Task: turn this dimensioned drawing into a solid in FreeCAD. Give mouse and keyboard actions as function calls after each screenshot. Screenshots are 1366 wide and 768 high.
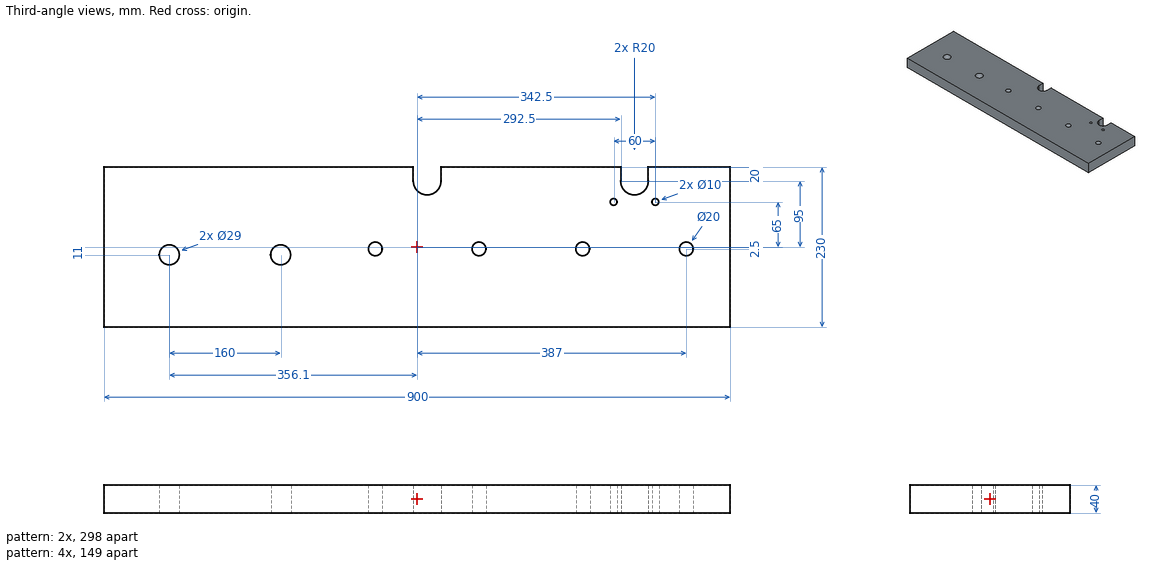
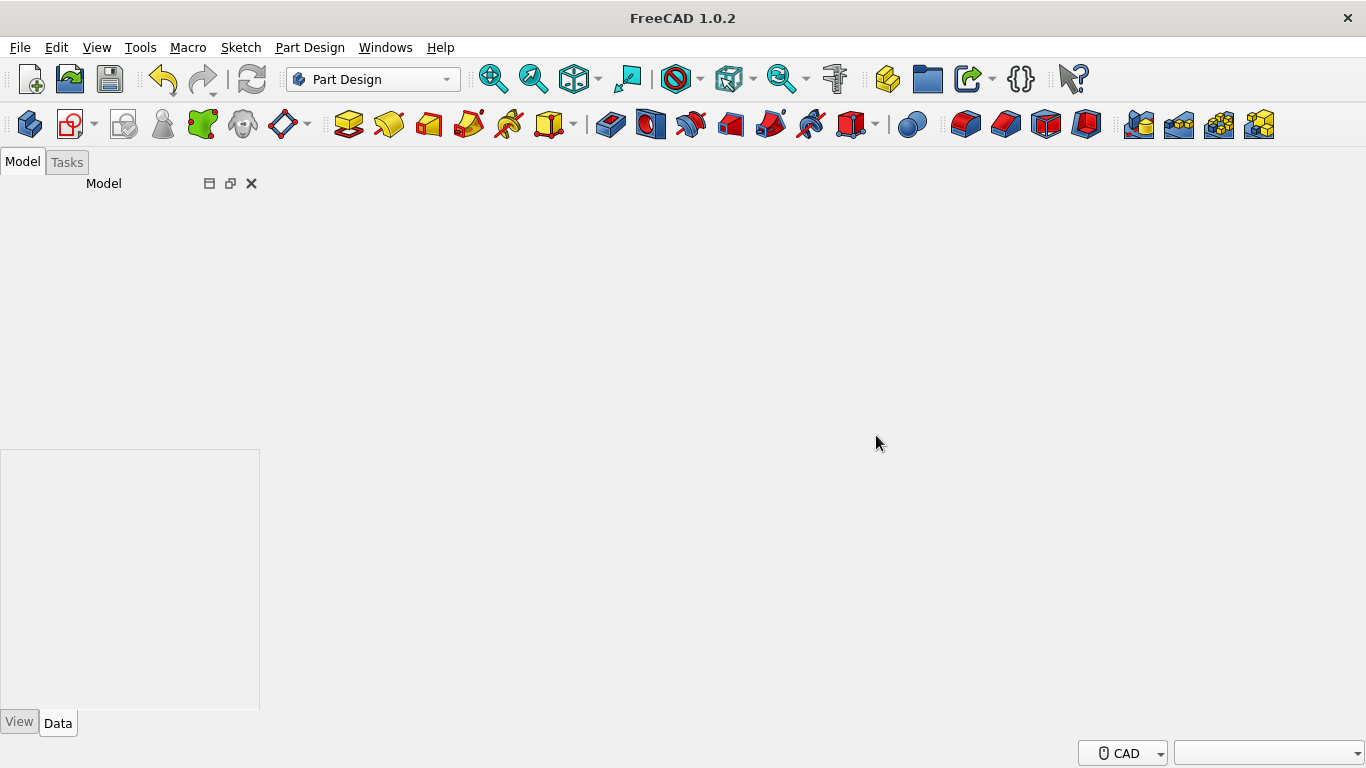
click(30, 80)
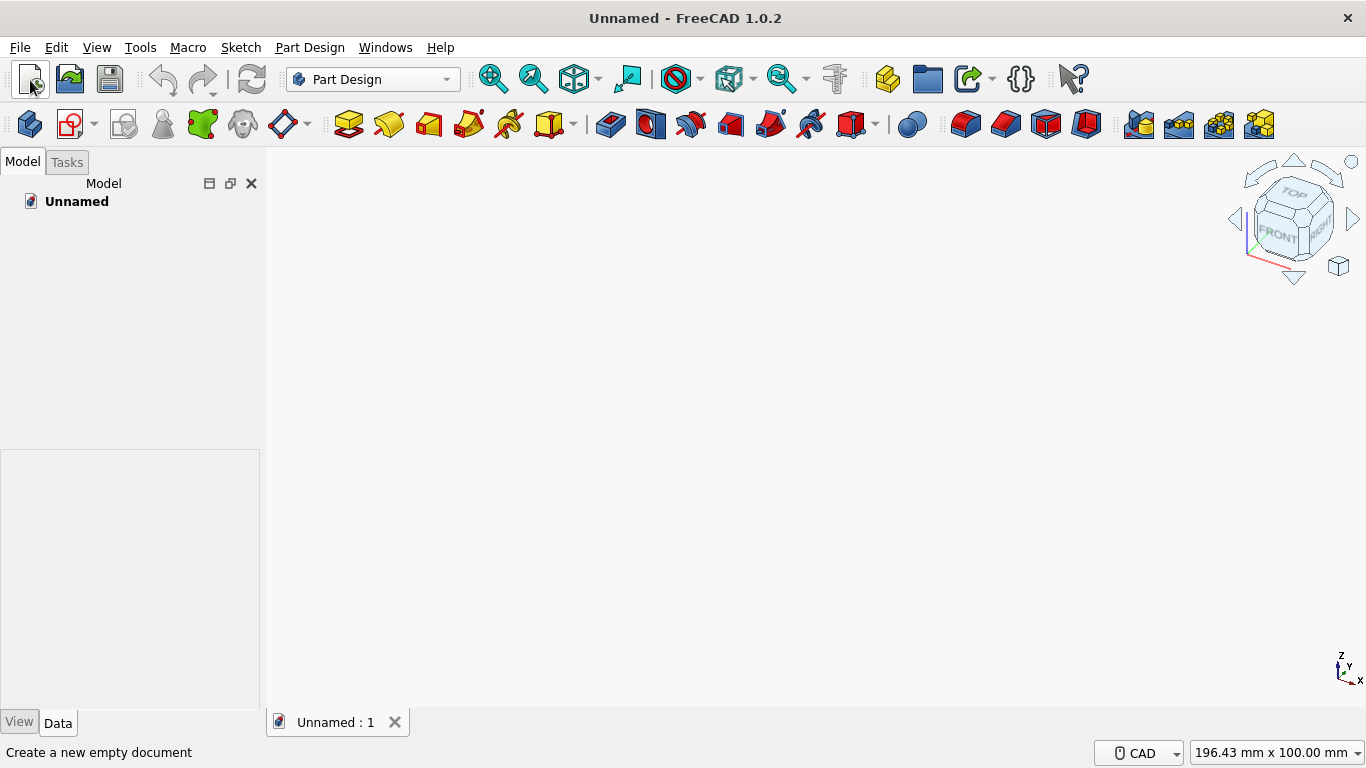
click(70, 124)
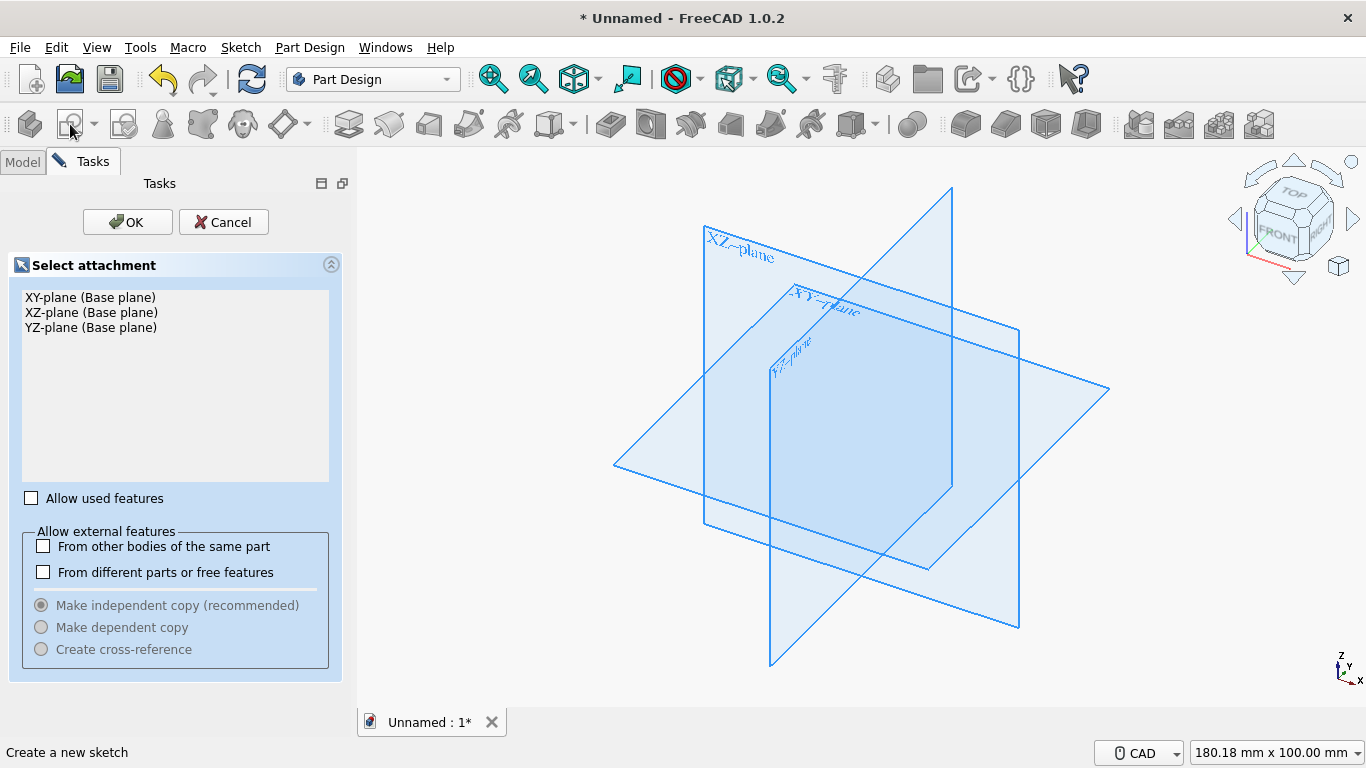
click(82, 298)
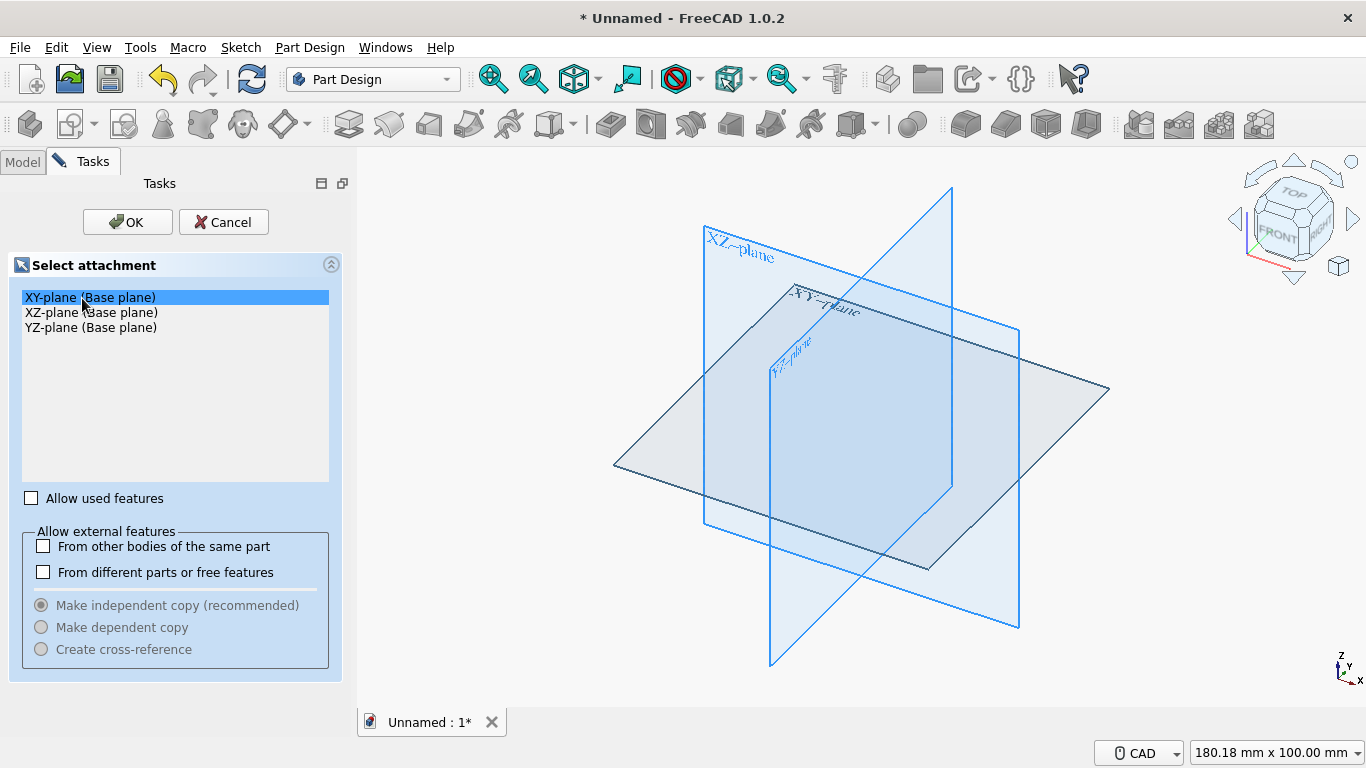
click(128, 222)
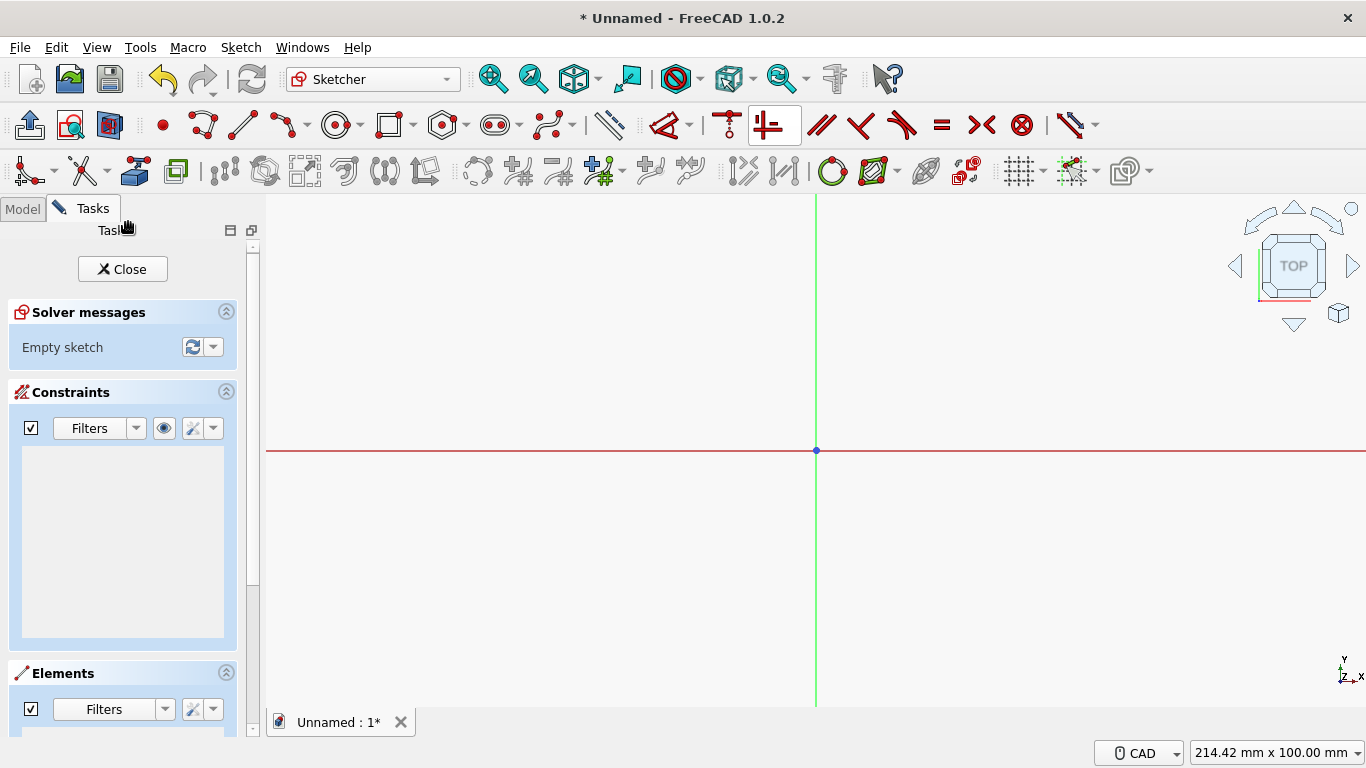
scroll(737, 450, down, 10)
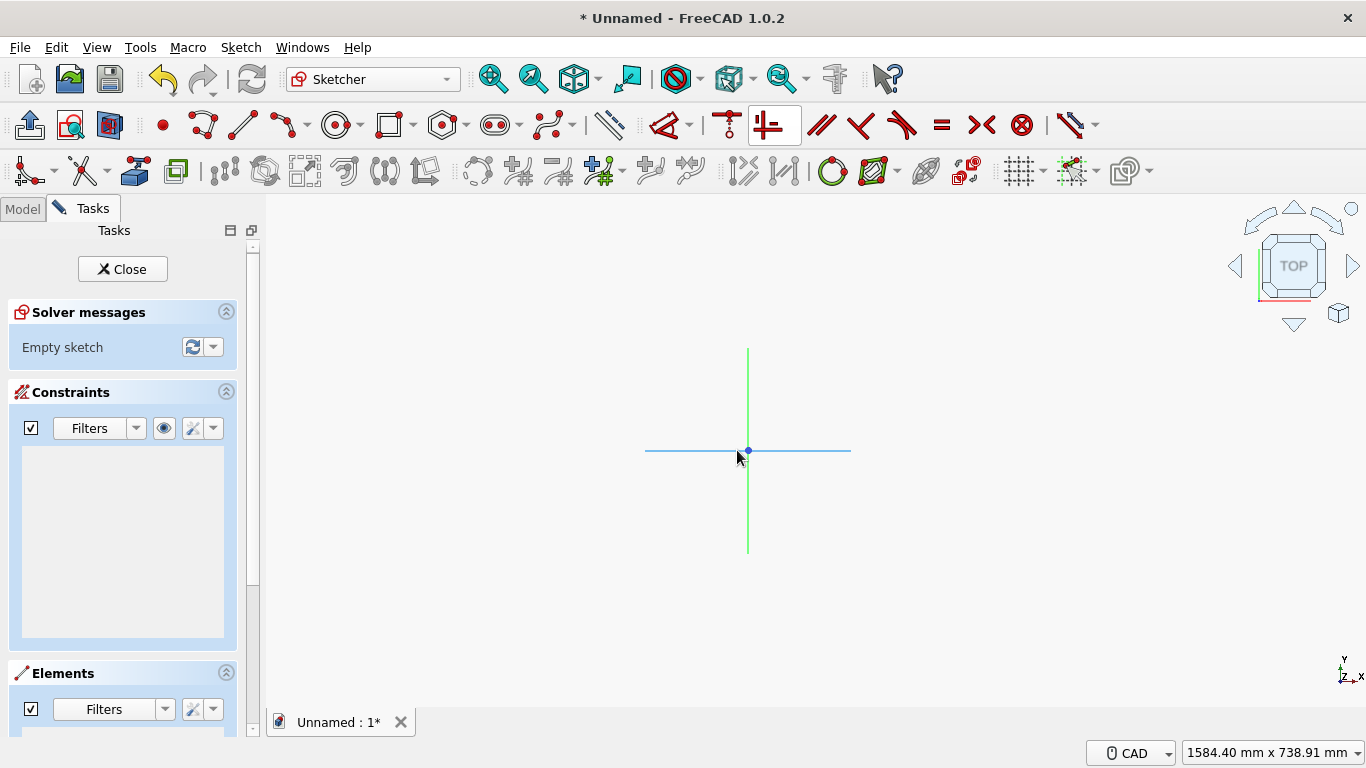
key(g)
key(v)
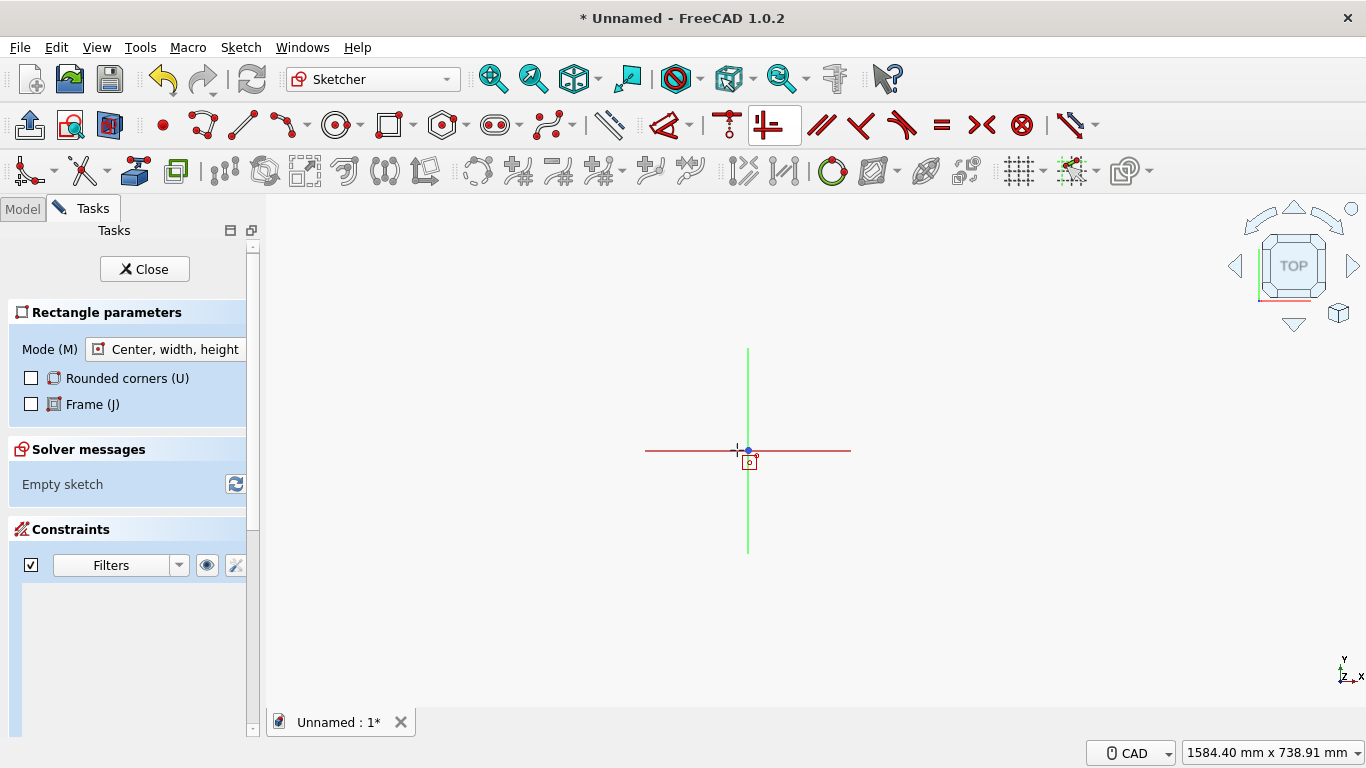
click(748, 450)
move(1060, 371)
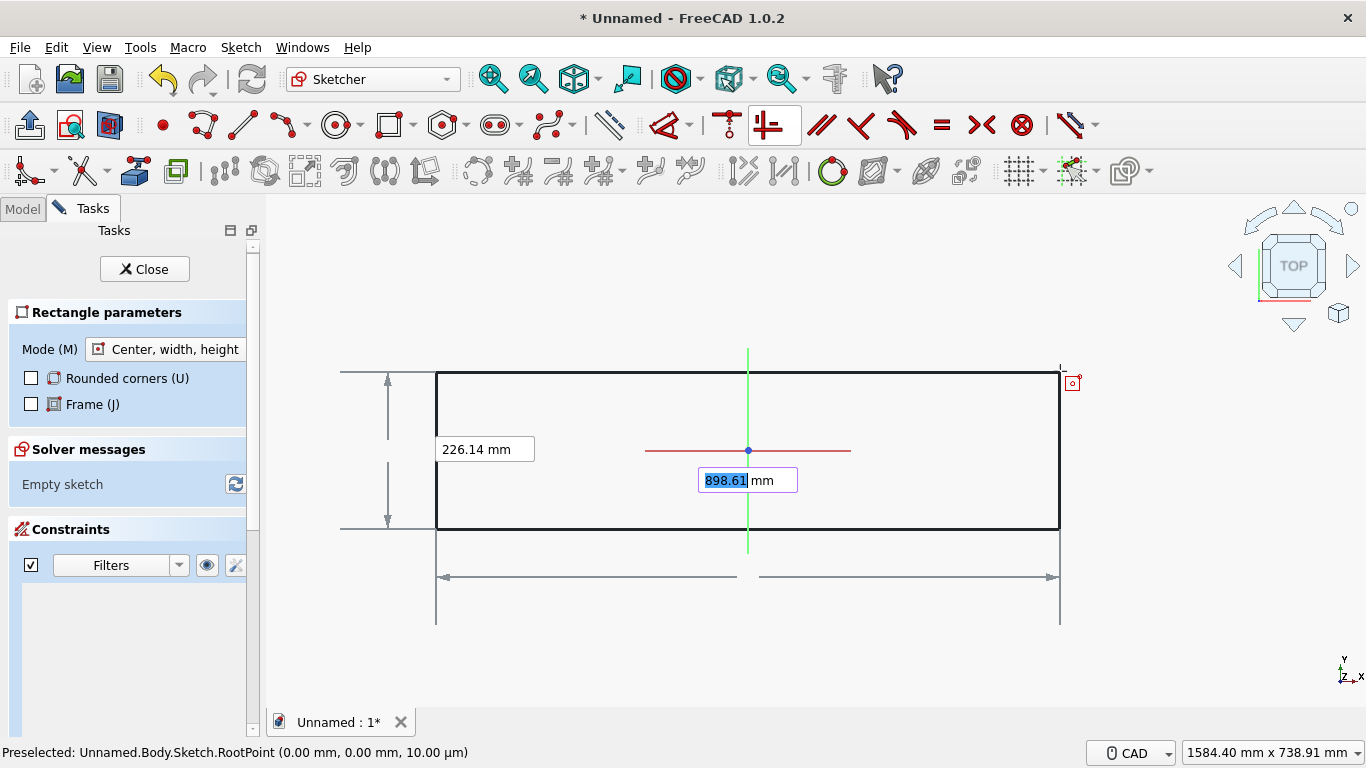
text(900)
key(Tab)
text(230)
key(Return)
key(Escape)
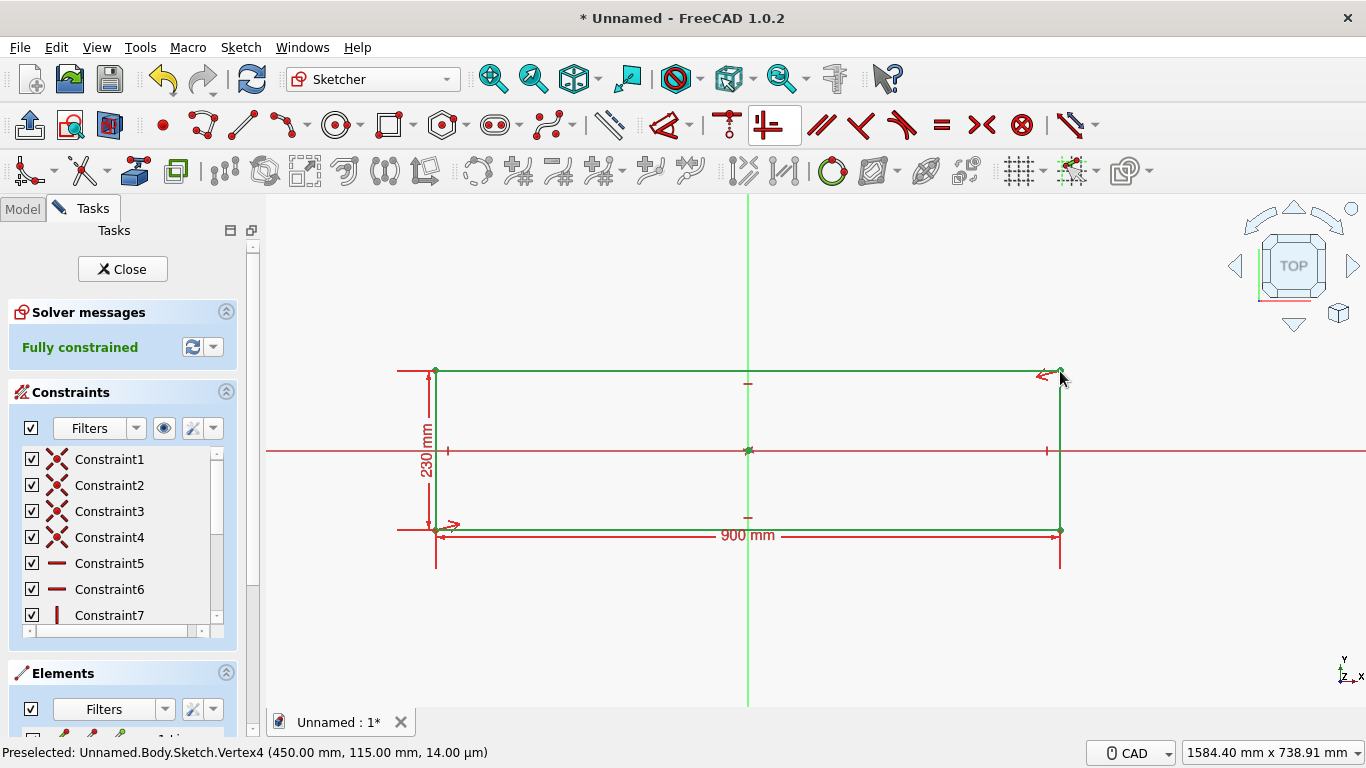
click(123, 269)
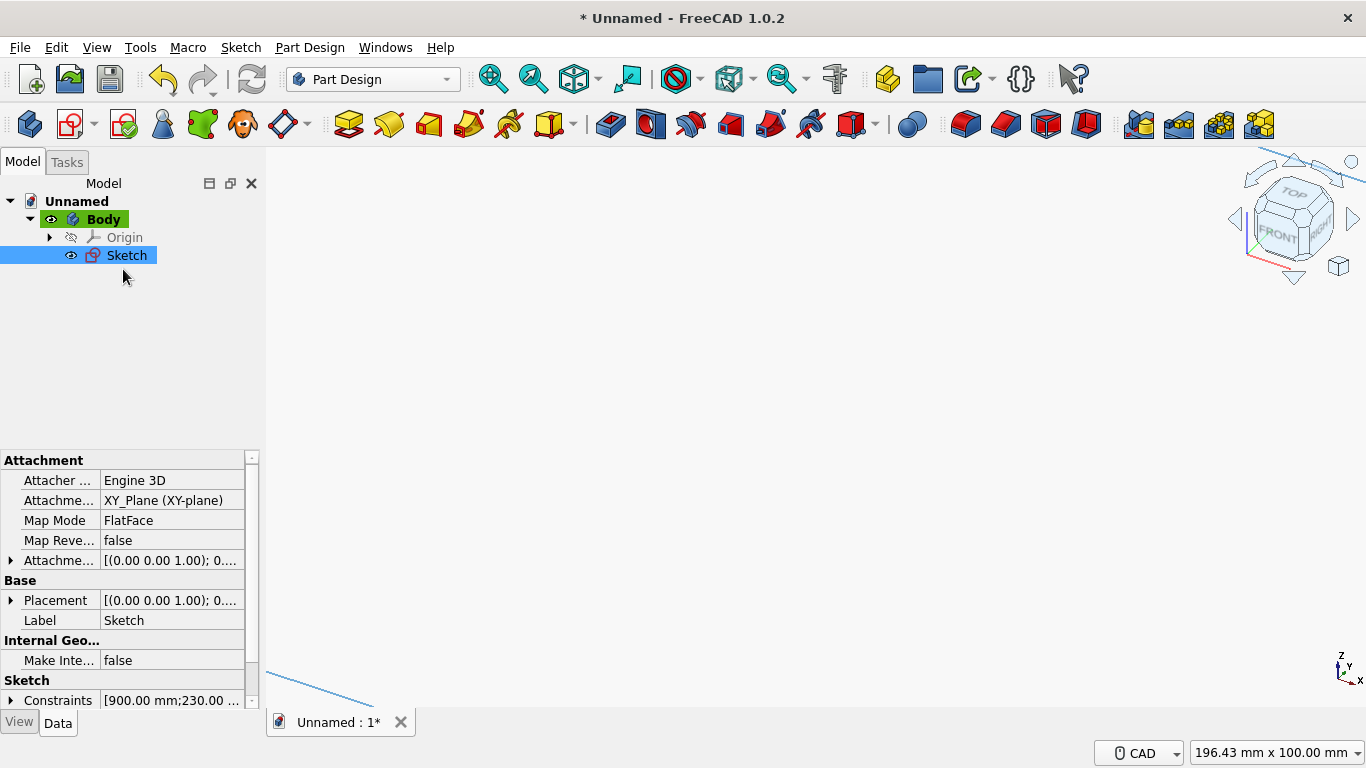
click(350, 124)